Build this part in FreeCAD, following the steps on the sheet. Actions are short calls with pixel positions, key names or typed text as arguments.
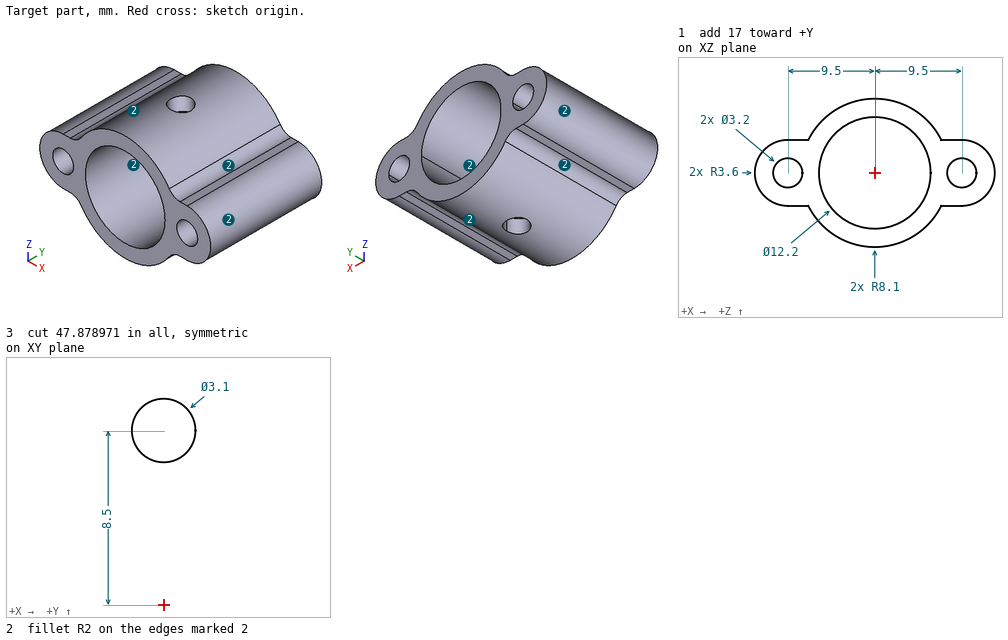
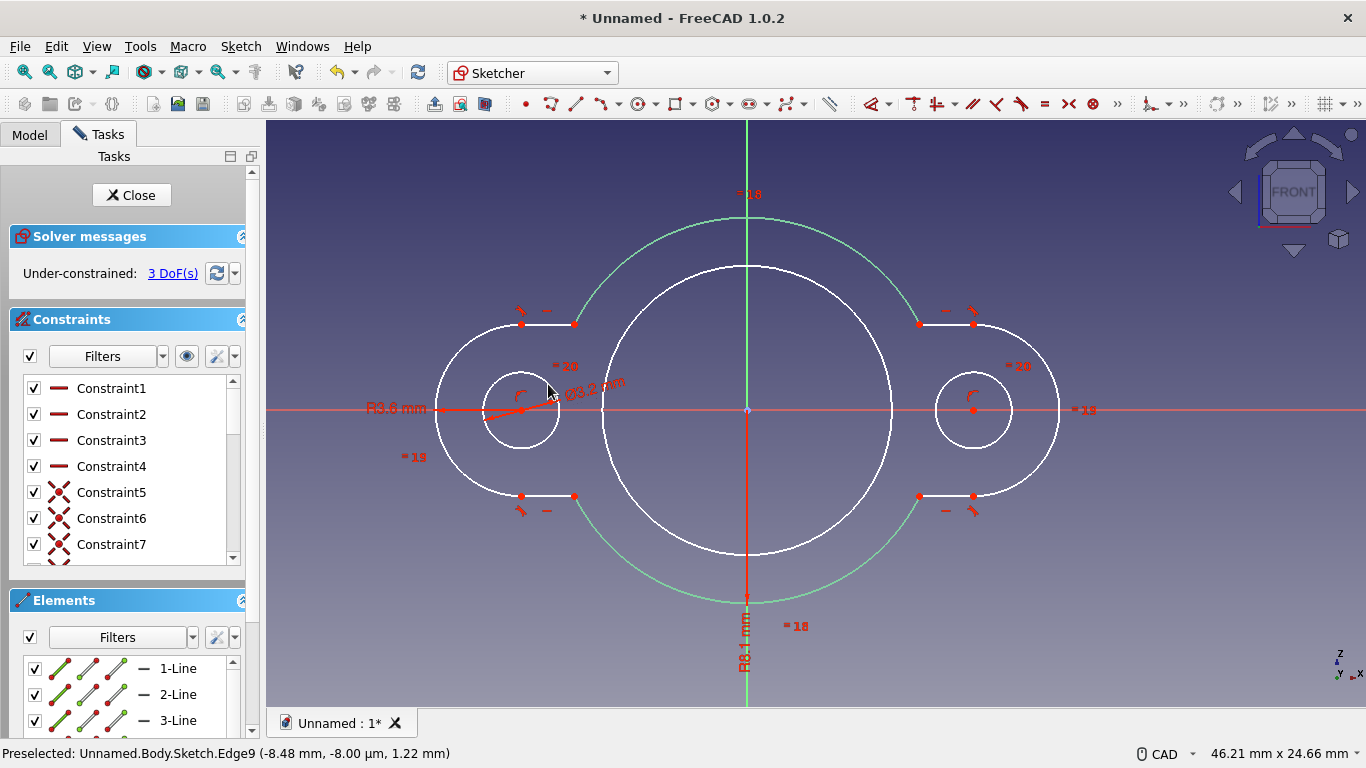
click(849, 308)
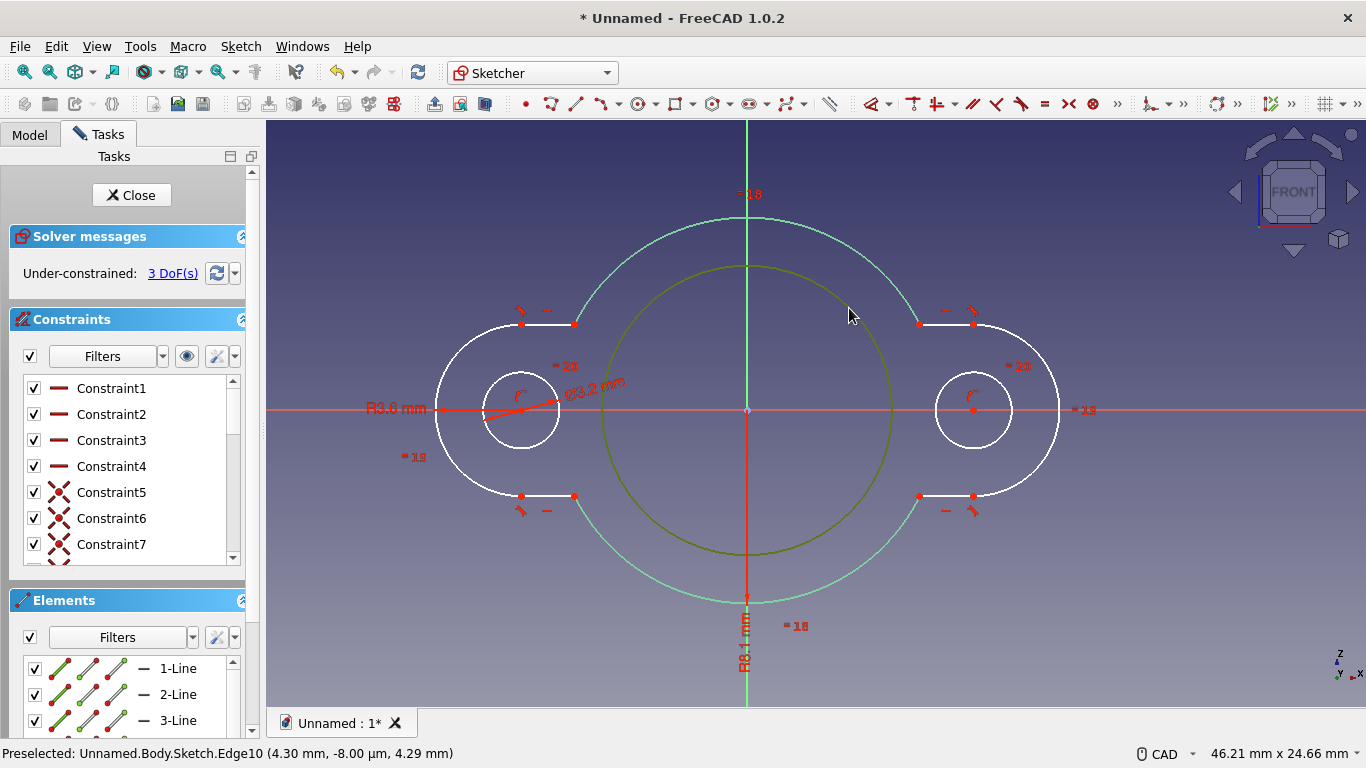
key(k)
key(o)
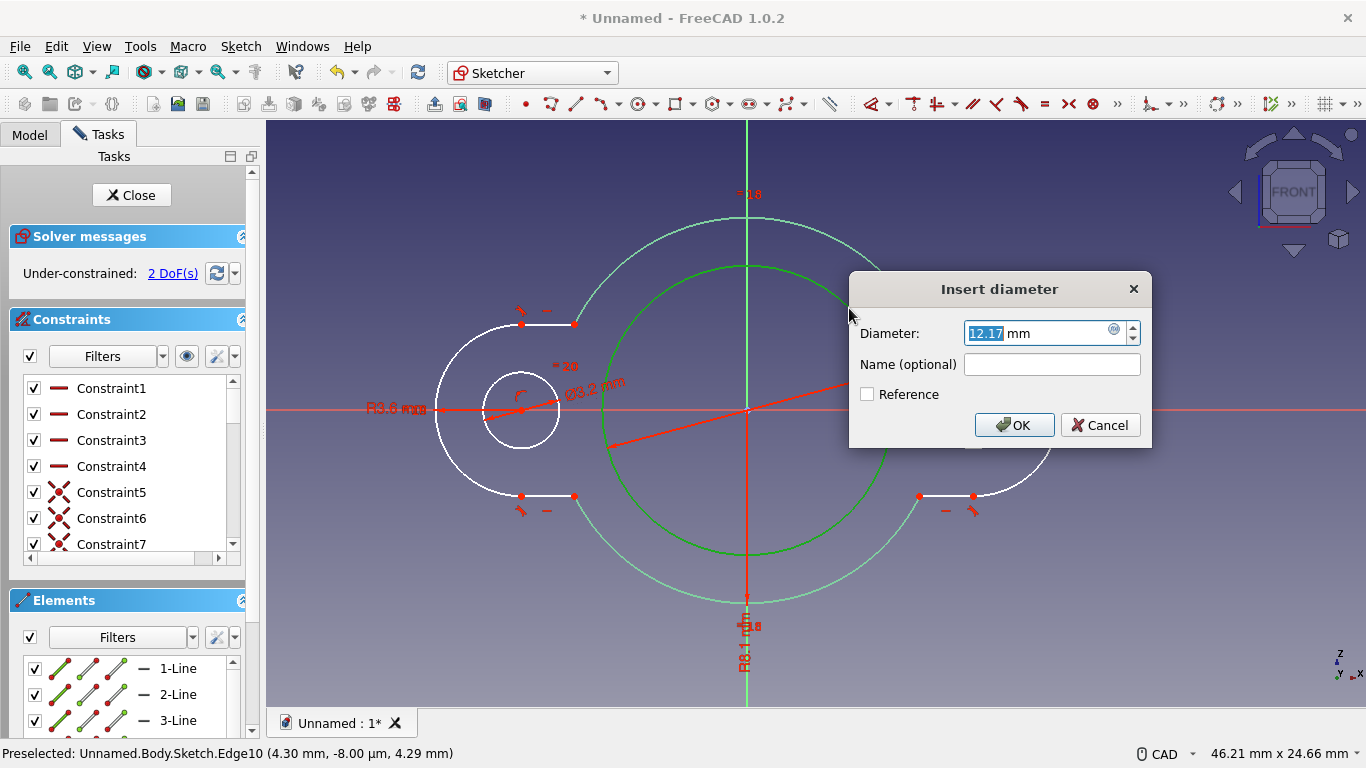
text(12.2)
key(Return)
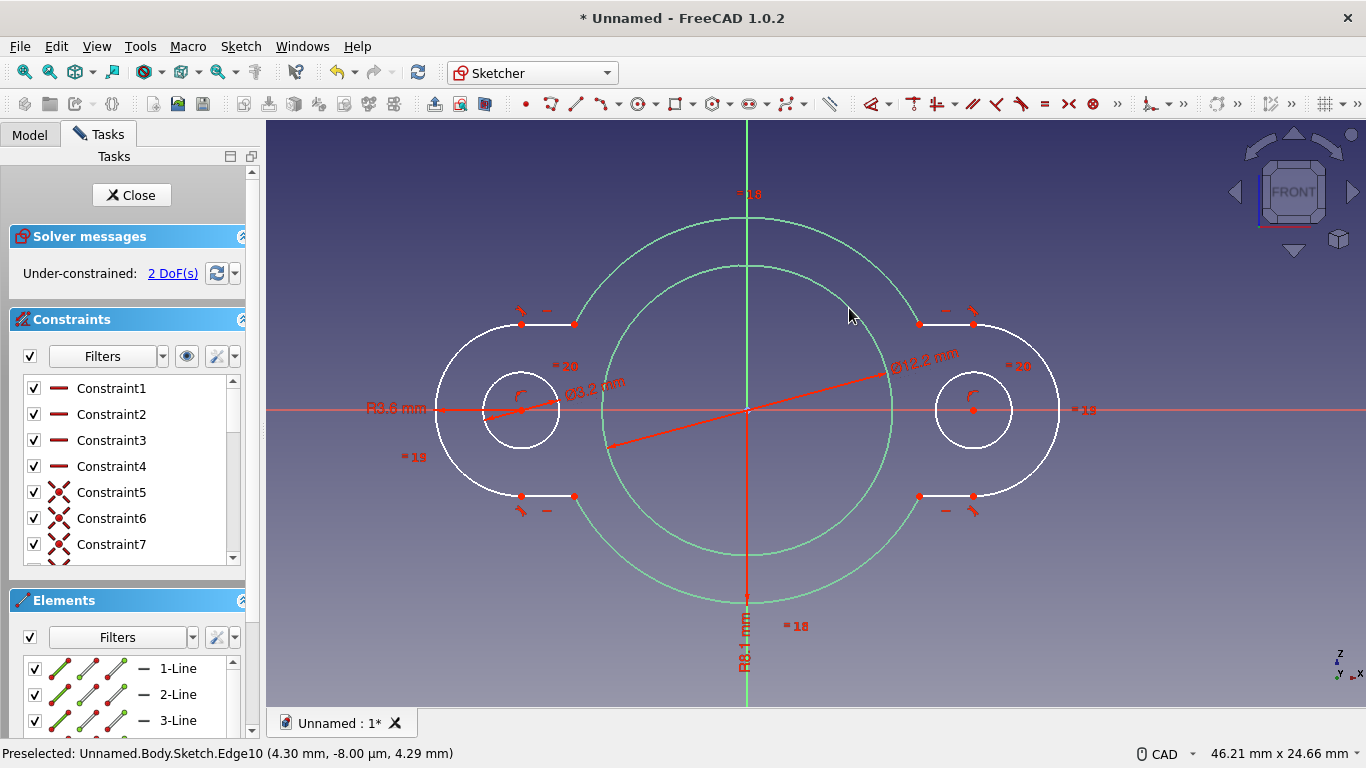
click(521, 410)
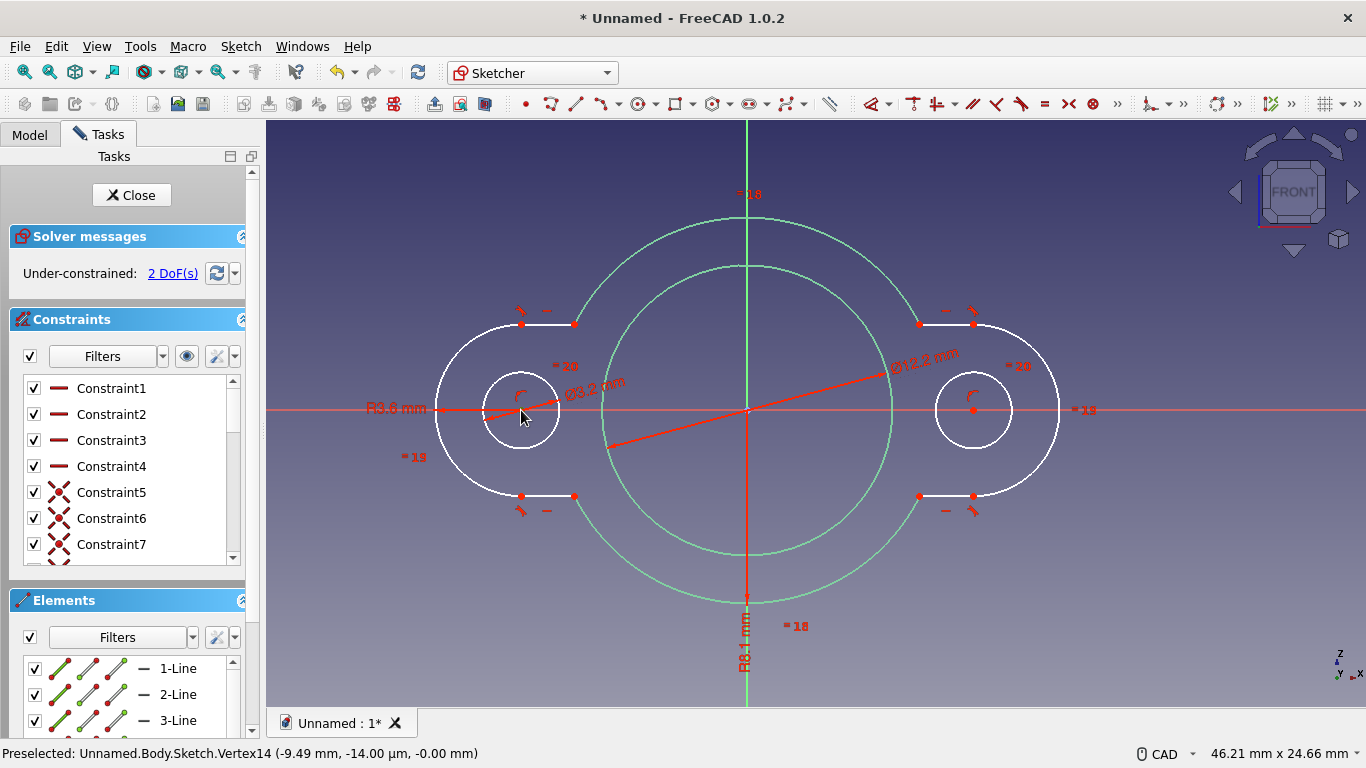
key(l)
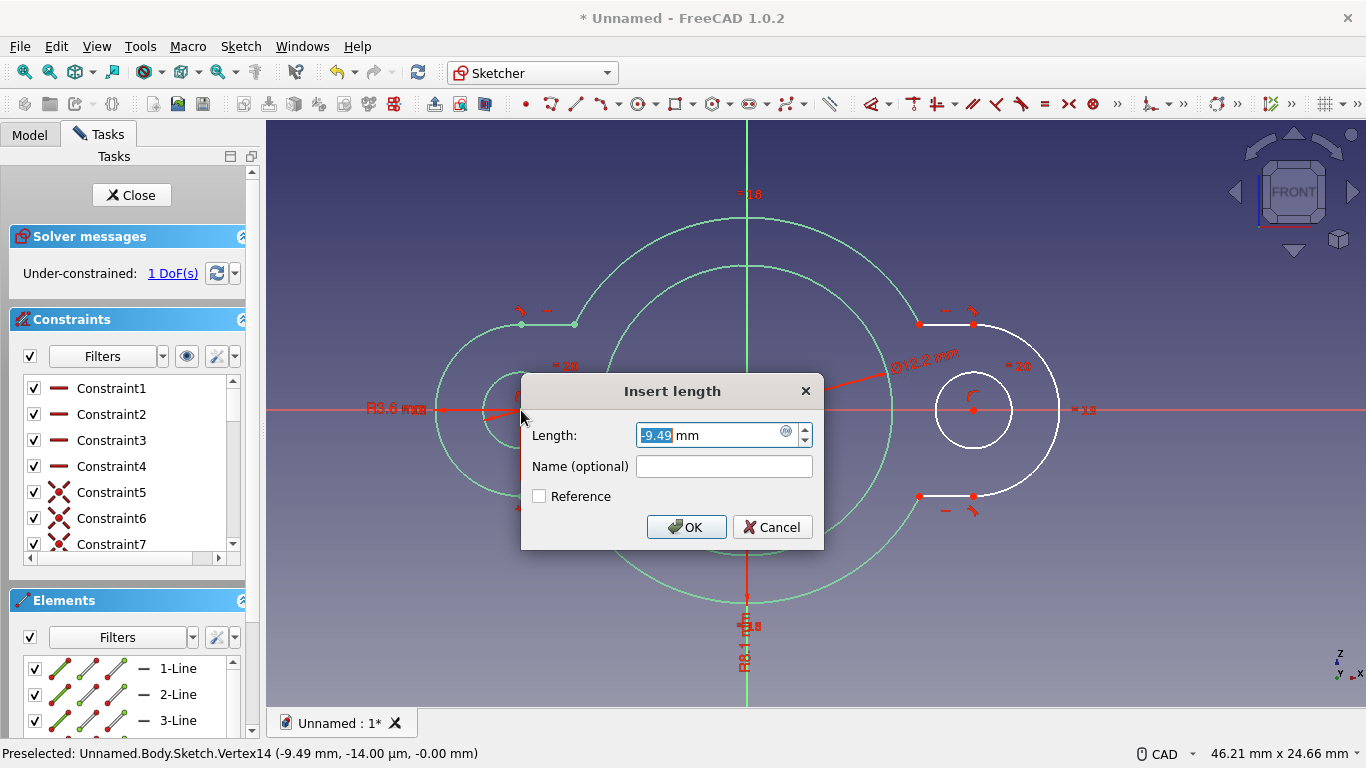
text(-9.5)
key(Return)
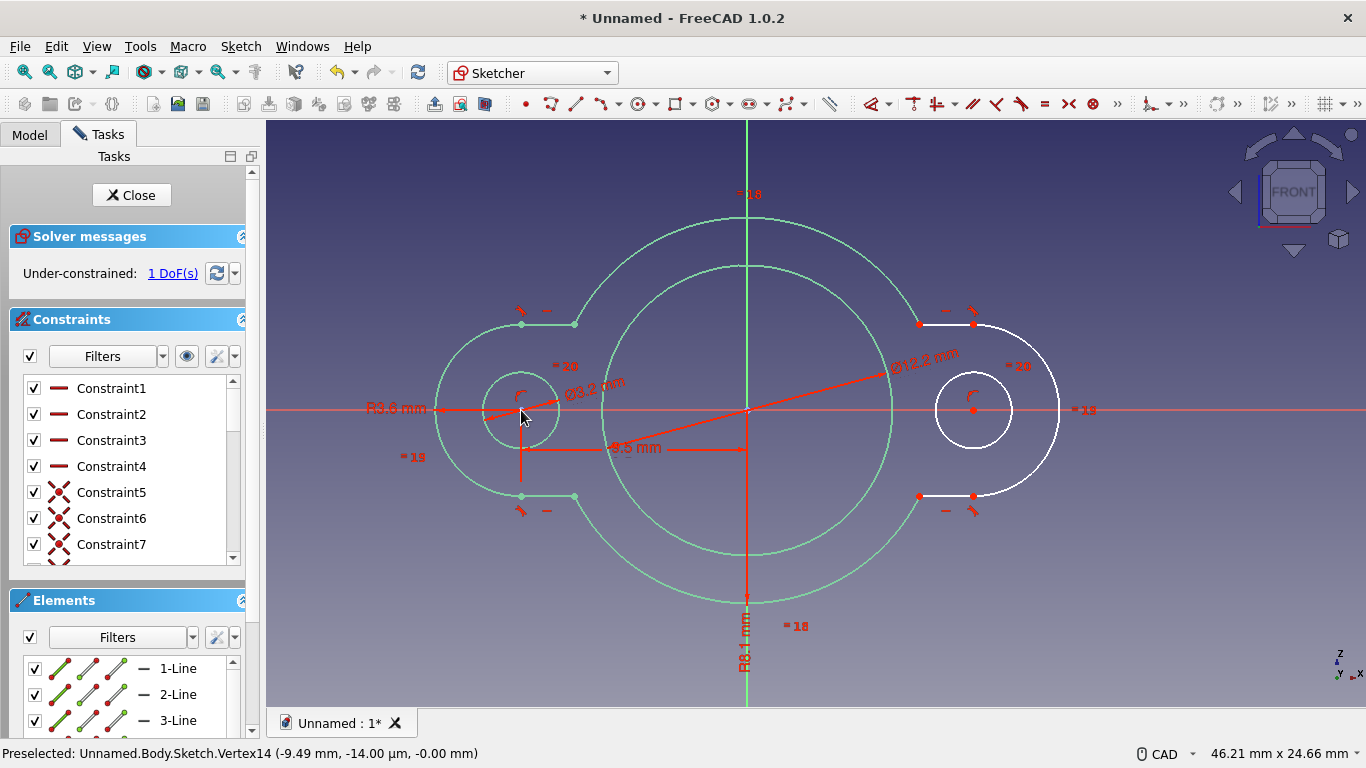
click(974, 410)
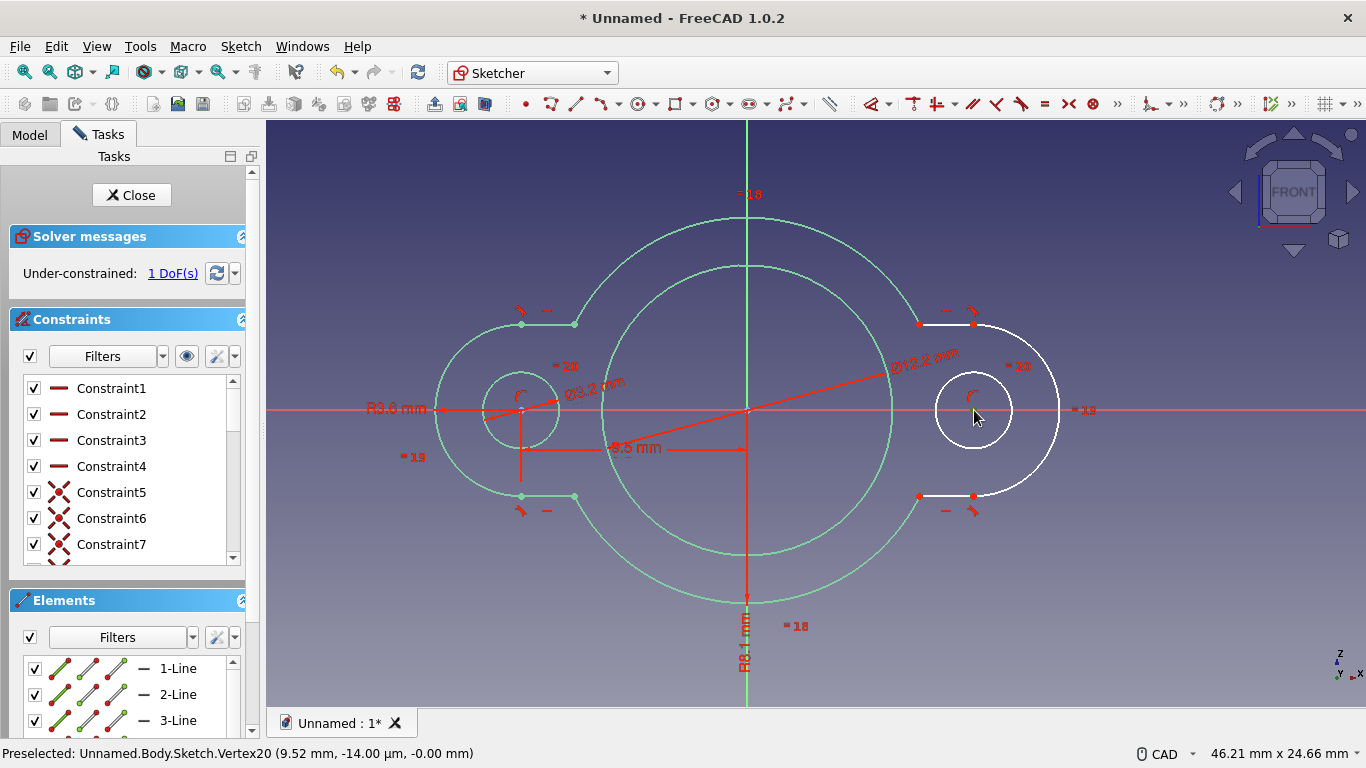
key(l)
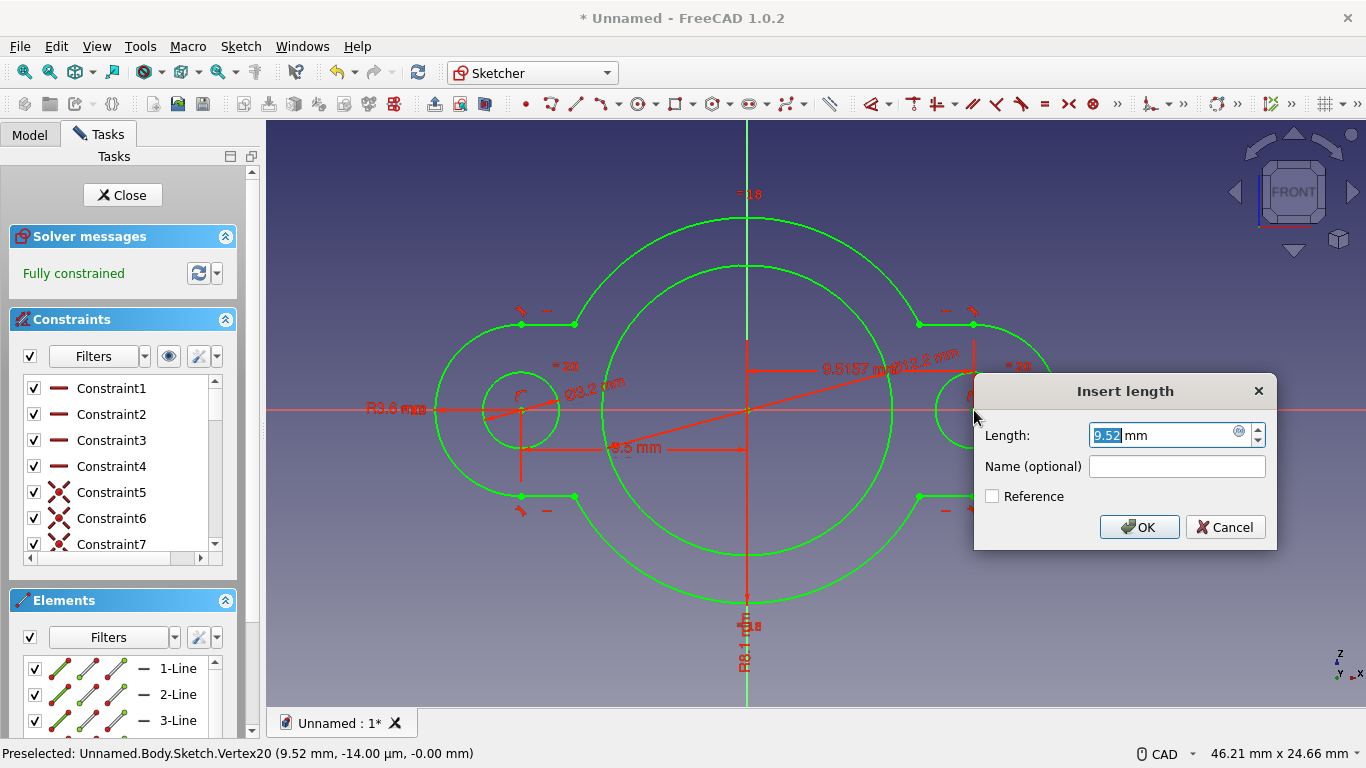
text(9.5)
key(Return)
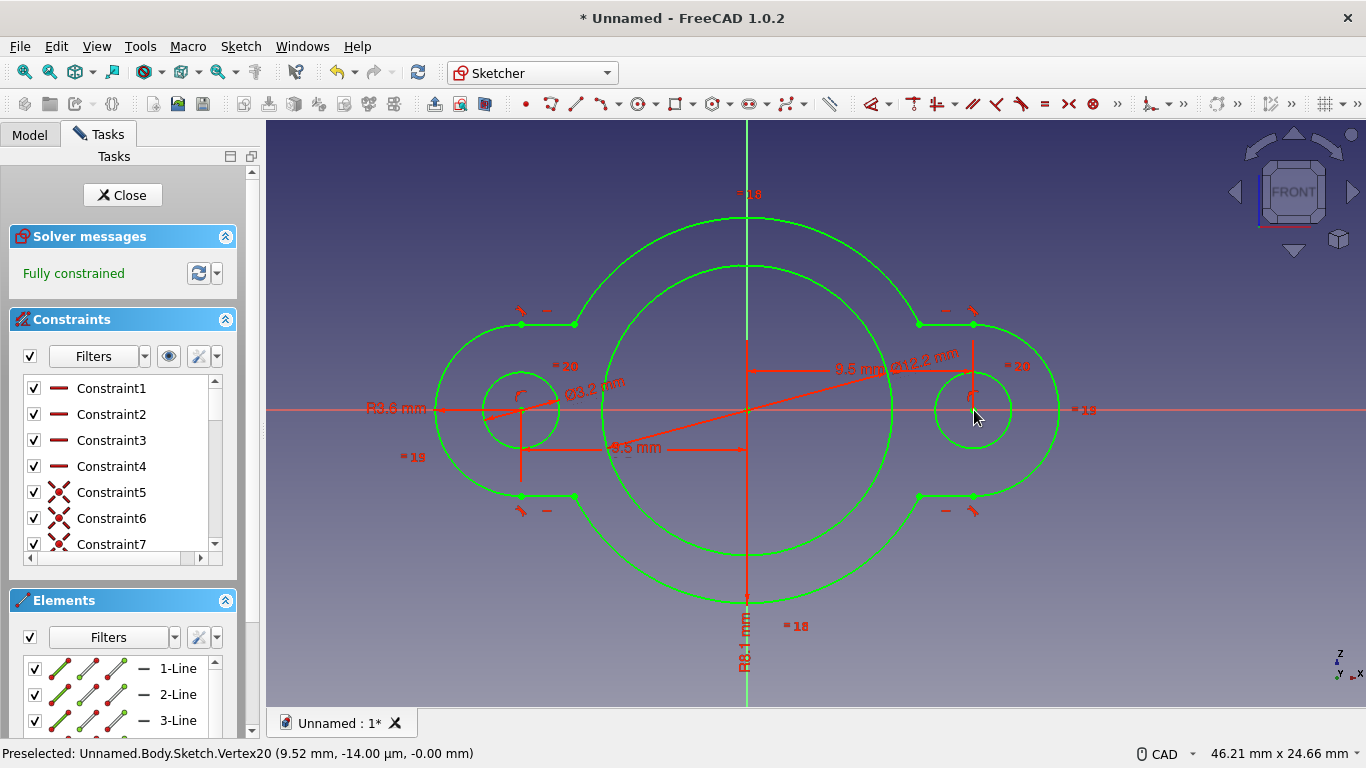
click(123, 195)